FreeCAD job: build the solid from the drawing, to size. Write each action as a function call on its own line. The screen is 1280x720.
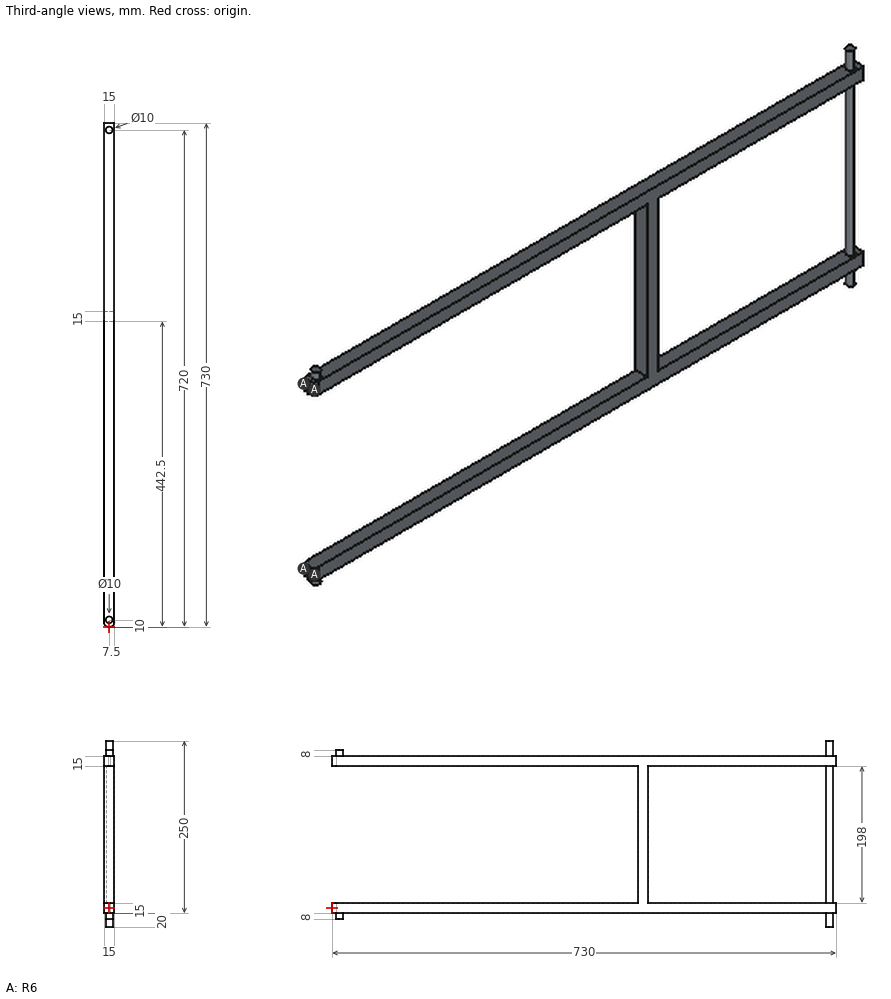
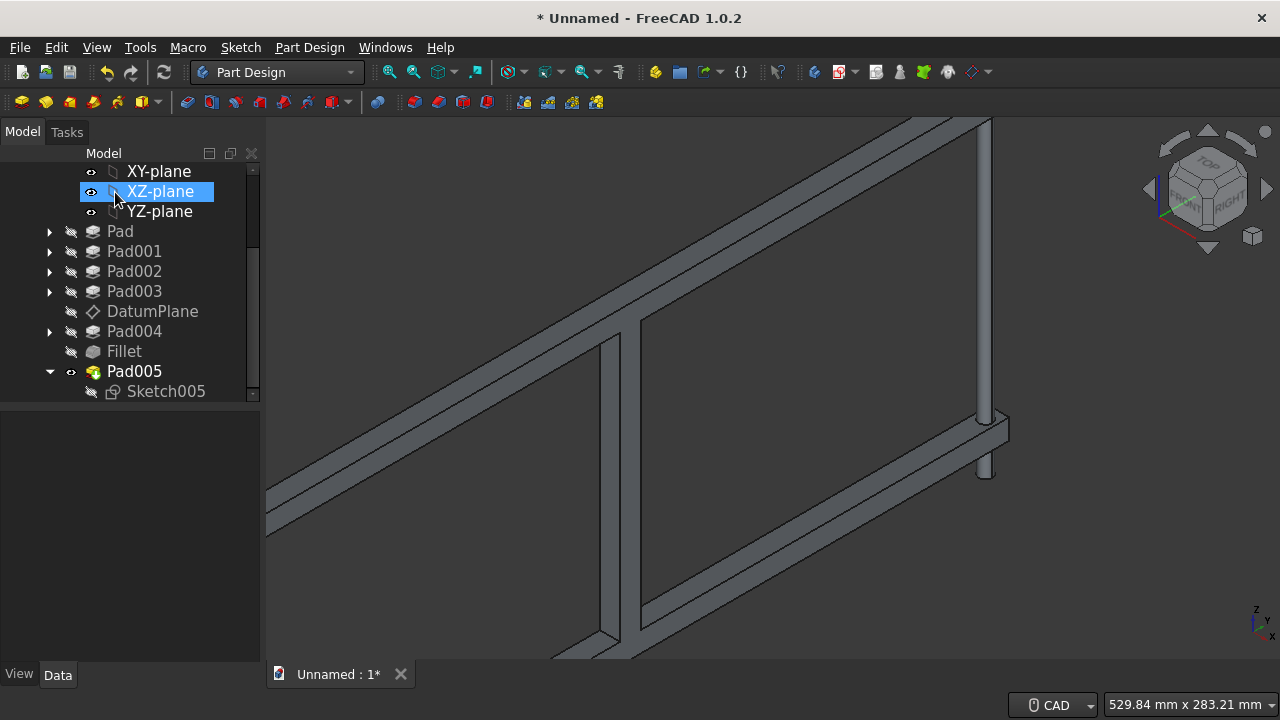
click(390, 72)